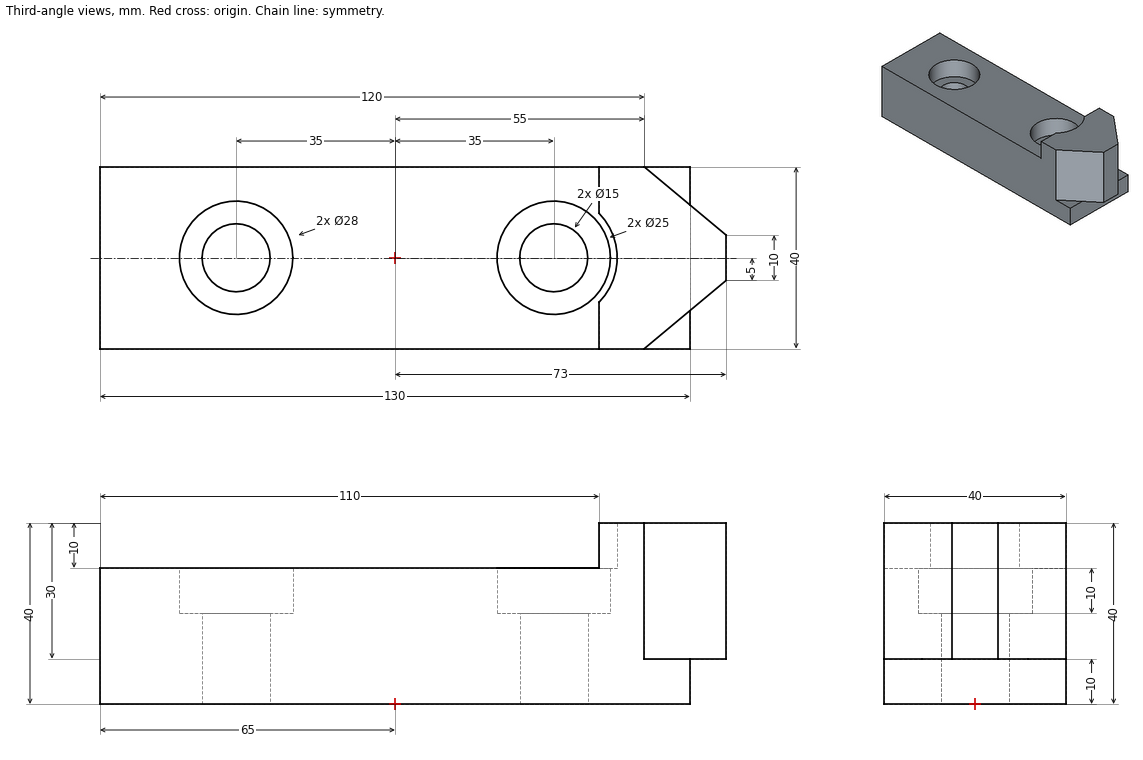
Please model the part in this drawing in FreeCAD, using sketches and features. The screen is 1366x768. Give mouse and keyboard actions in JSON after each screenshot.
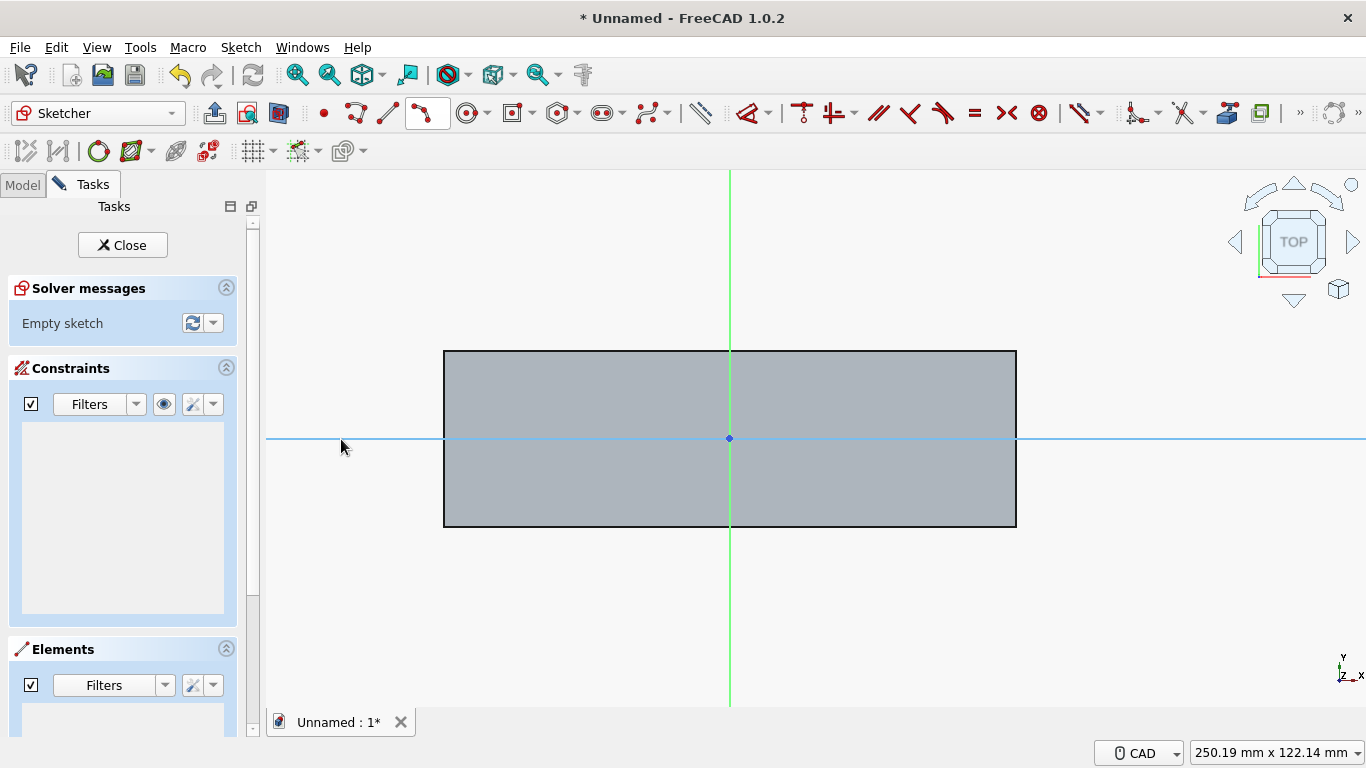
{"action": "left_click", "coordinate": [356, 114]}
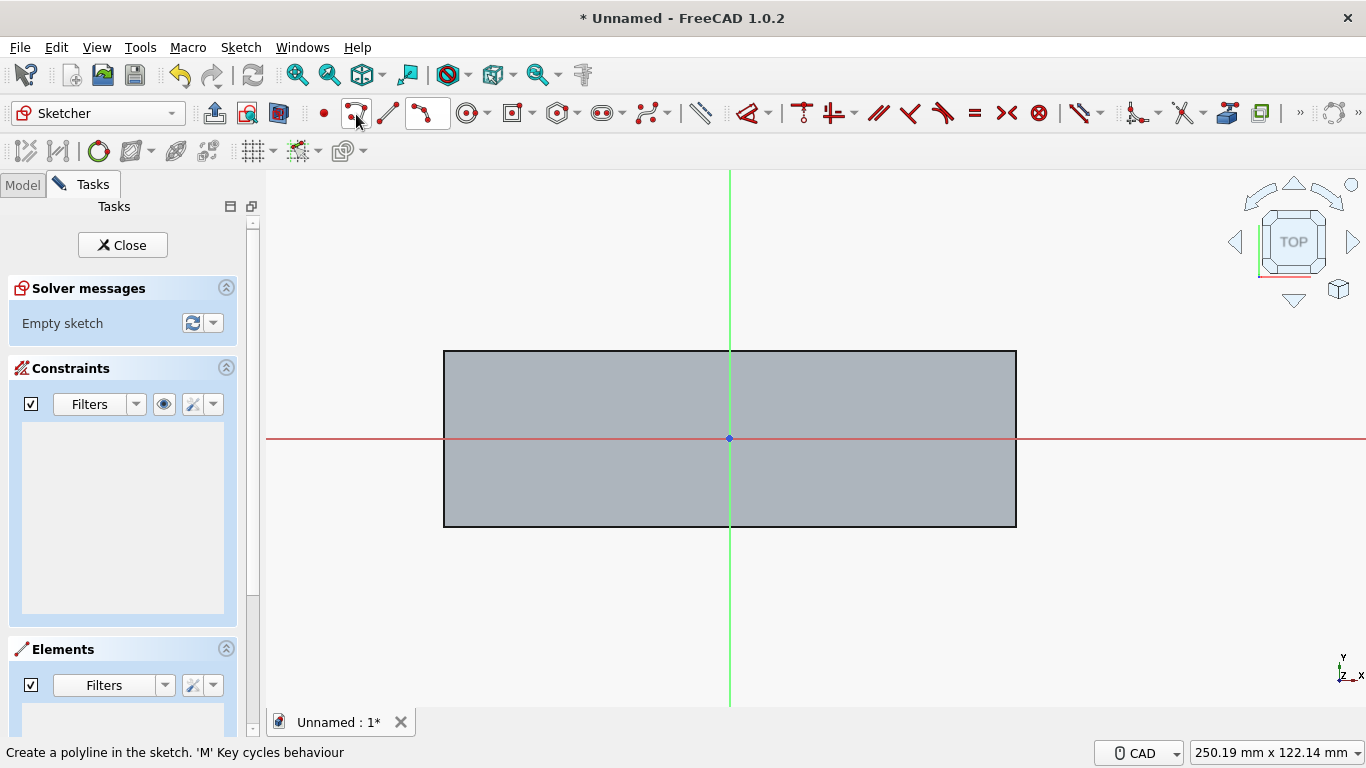
{"action": "left_click", "coordinate": [972, 351]}
{"action": "left_click", "coordinate": [444, 351]}
{"action": "left_click", "coordinate": [444, 527]}
{"action": "left_click", "coordinate": [972, 527]}
{"action": "left_click", "coordinate": [1051, 461]}
{"action": "left_click", "coordinate": [1051, 417]}
{"action": "left_click", "coordinate": [972, 352]}
{"action": "key", "text": "Escape"}
{"action": "key", "text": "Escape"}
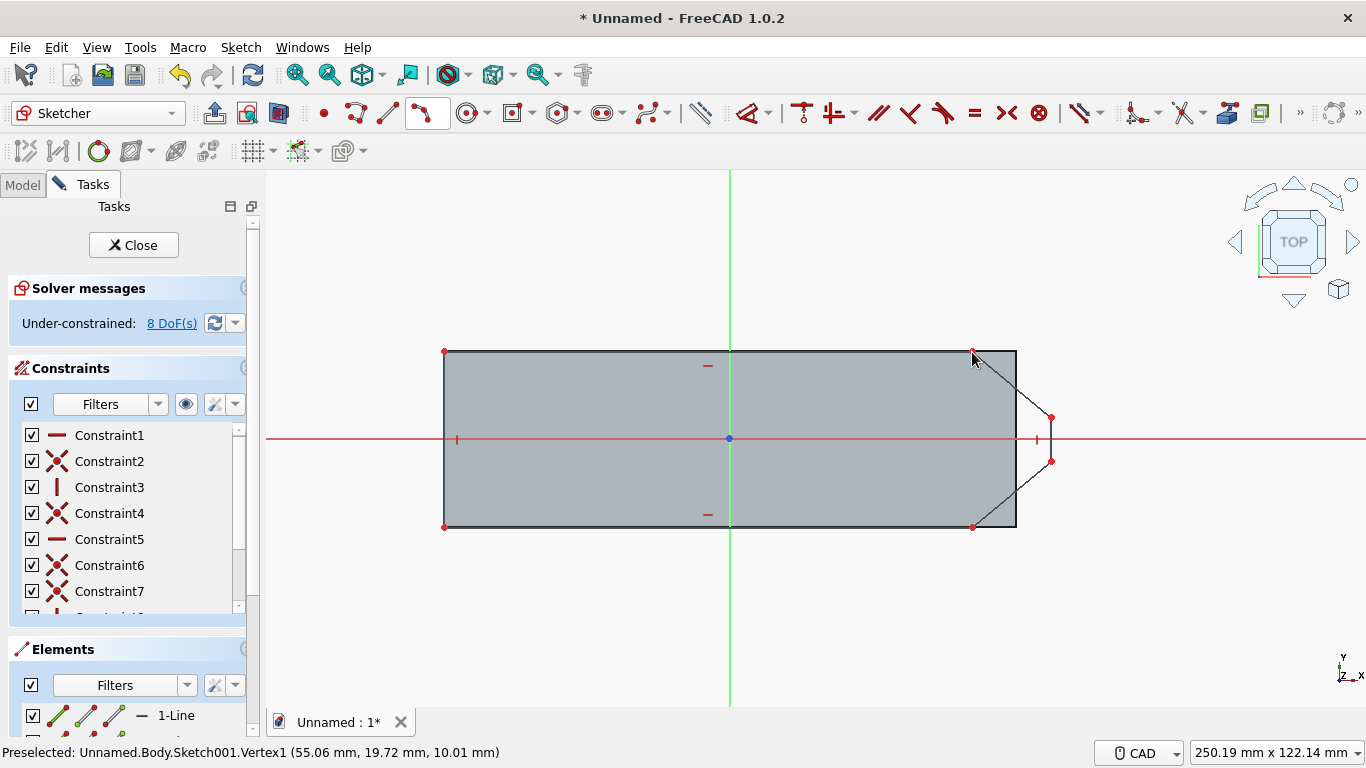
{"action": "left_click", "coordinate": [972, 352]}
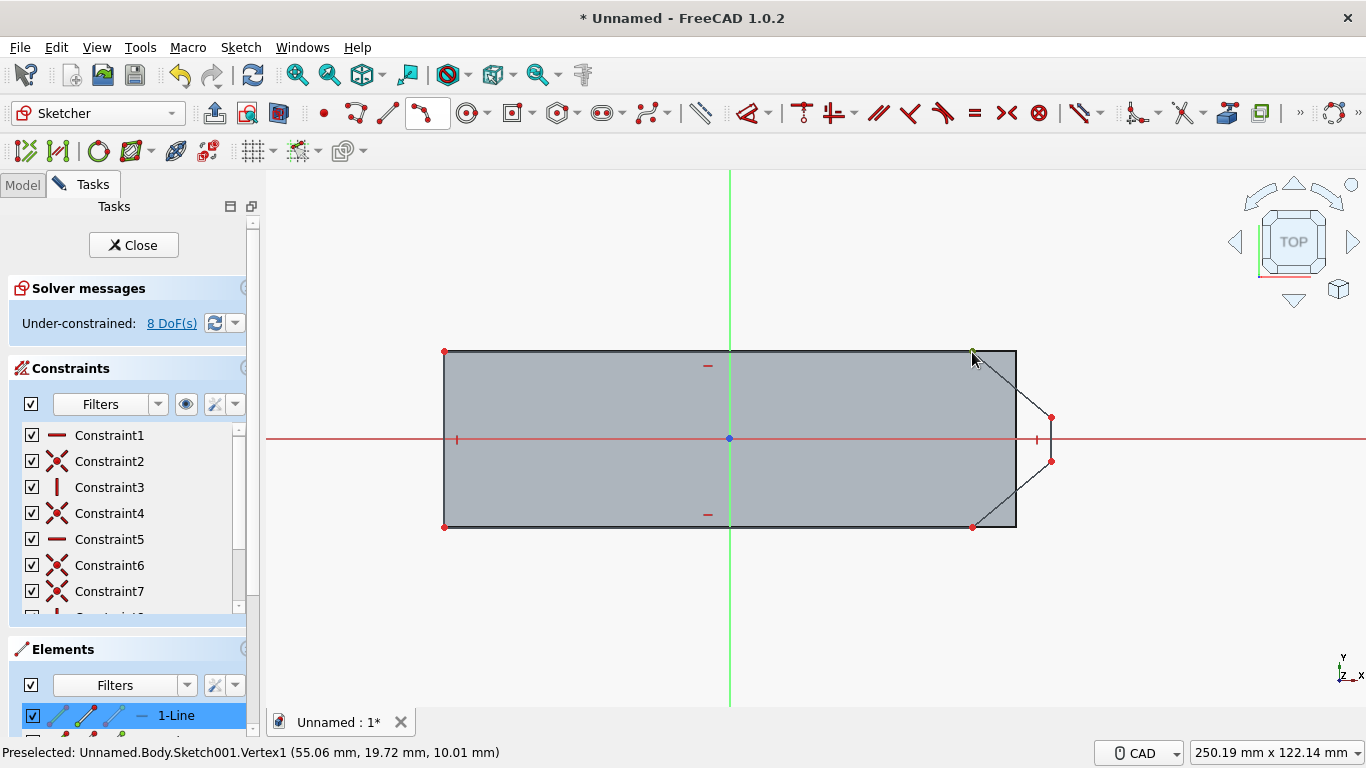
{"action": "left_click", "coordinate": [972, 528]}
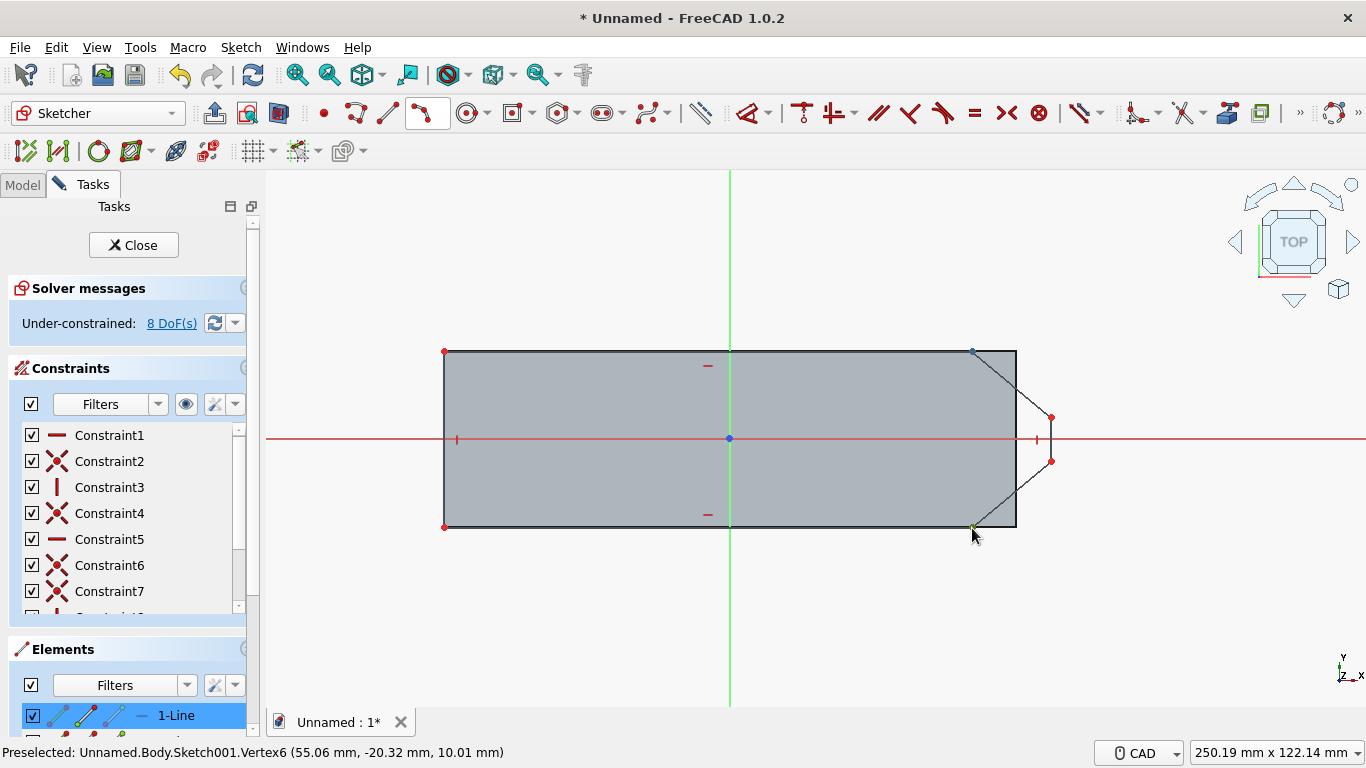
{"action": "left_click", "coordinate": [359, 439]}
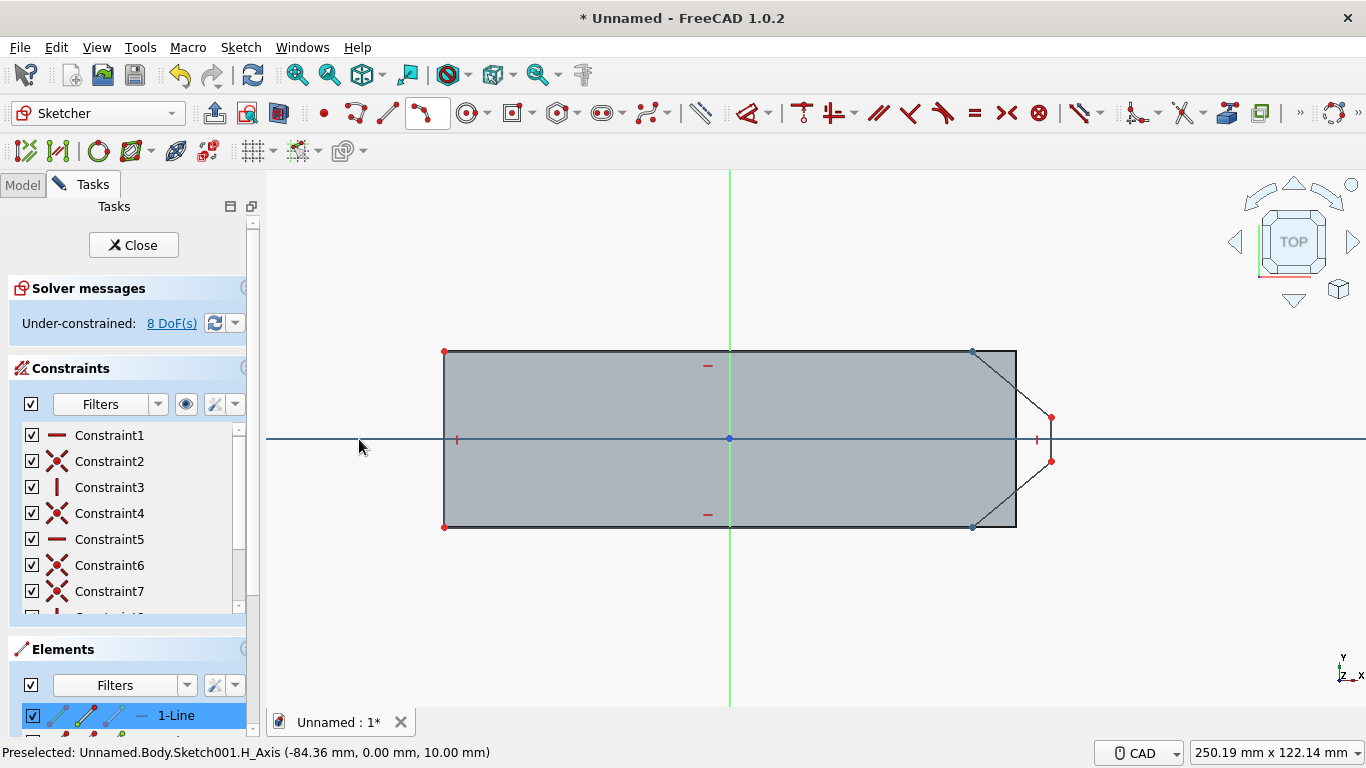
{"action": "left_click", "coordinate": [1008, 114]}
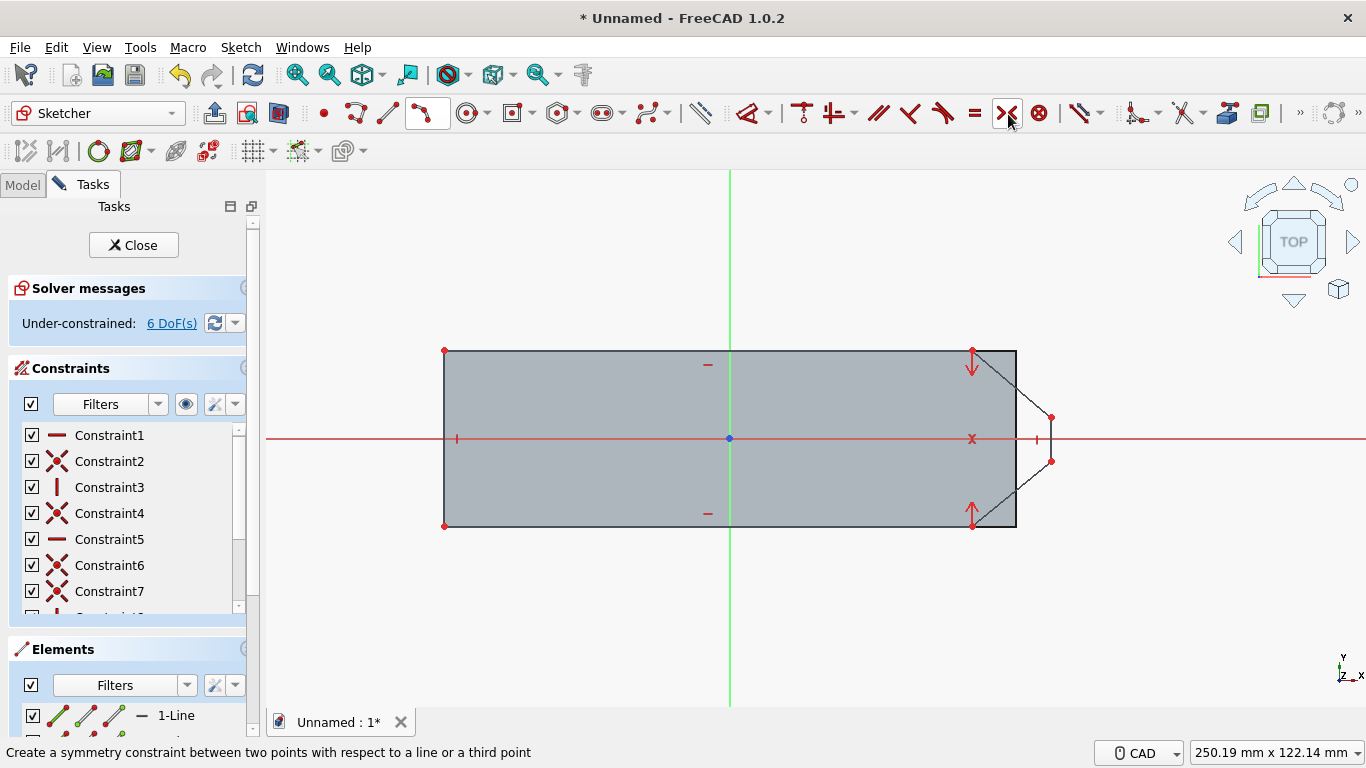
{"action": "left_click", "coordinate": [748, 114]}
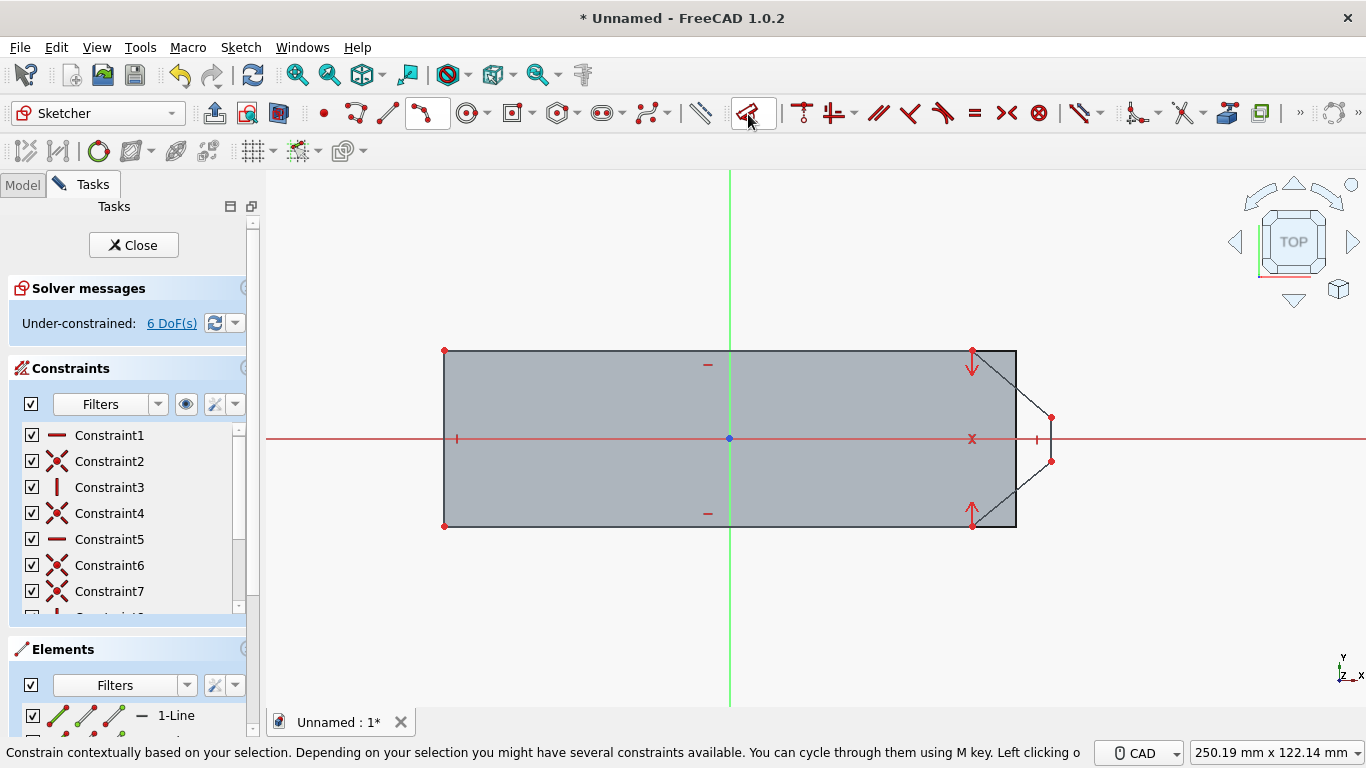
{"action": "left_click", "coordinate": [444, 404]}
{"action": "left_click", "coordinate": [410, 398]}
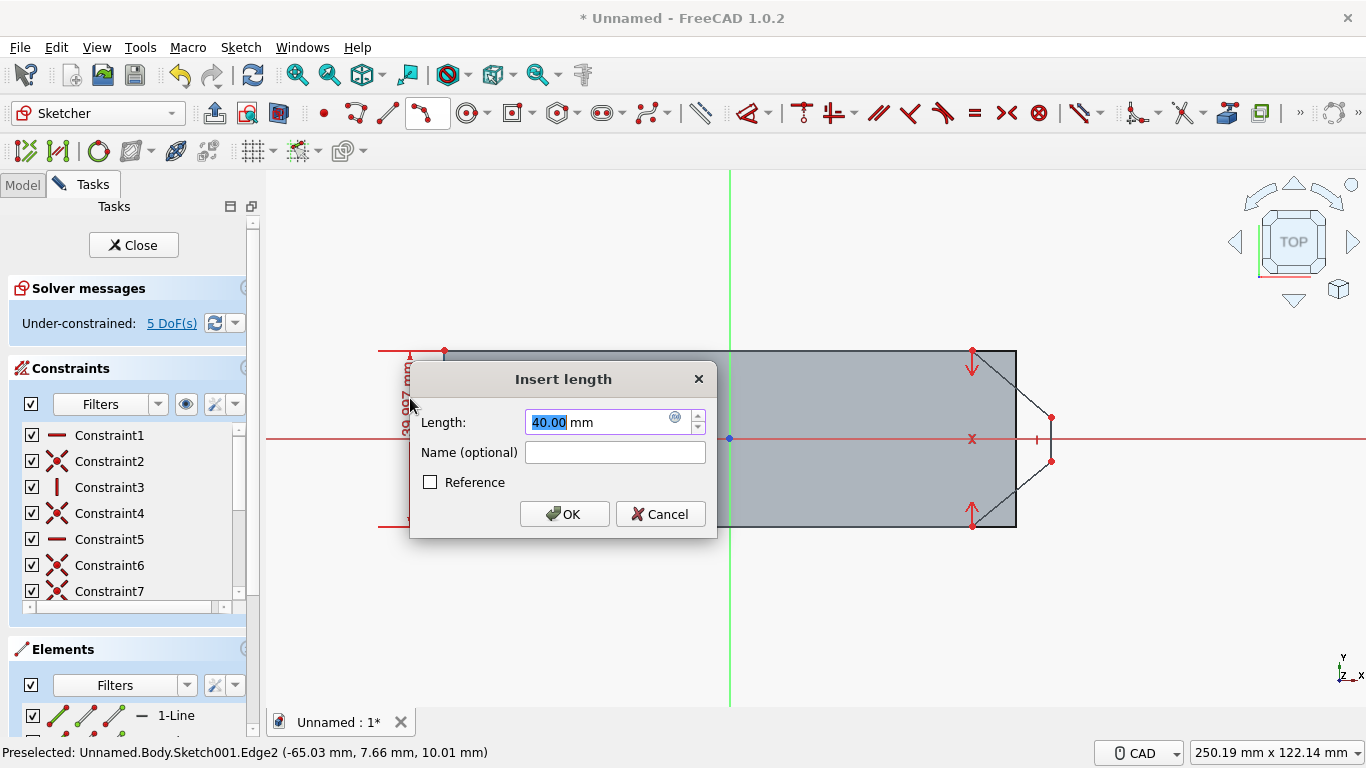
{"action": "type", "text": "40"}
{"action": "key", "text": "Return"}